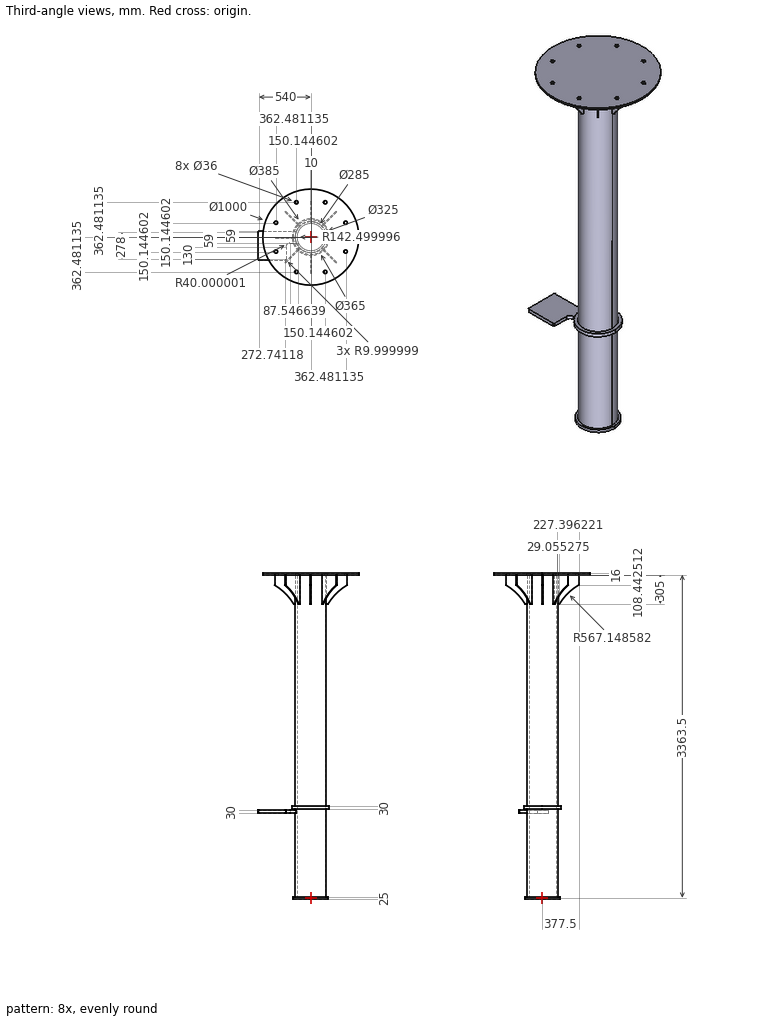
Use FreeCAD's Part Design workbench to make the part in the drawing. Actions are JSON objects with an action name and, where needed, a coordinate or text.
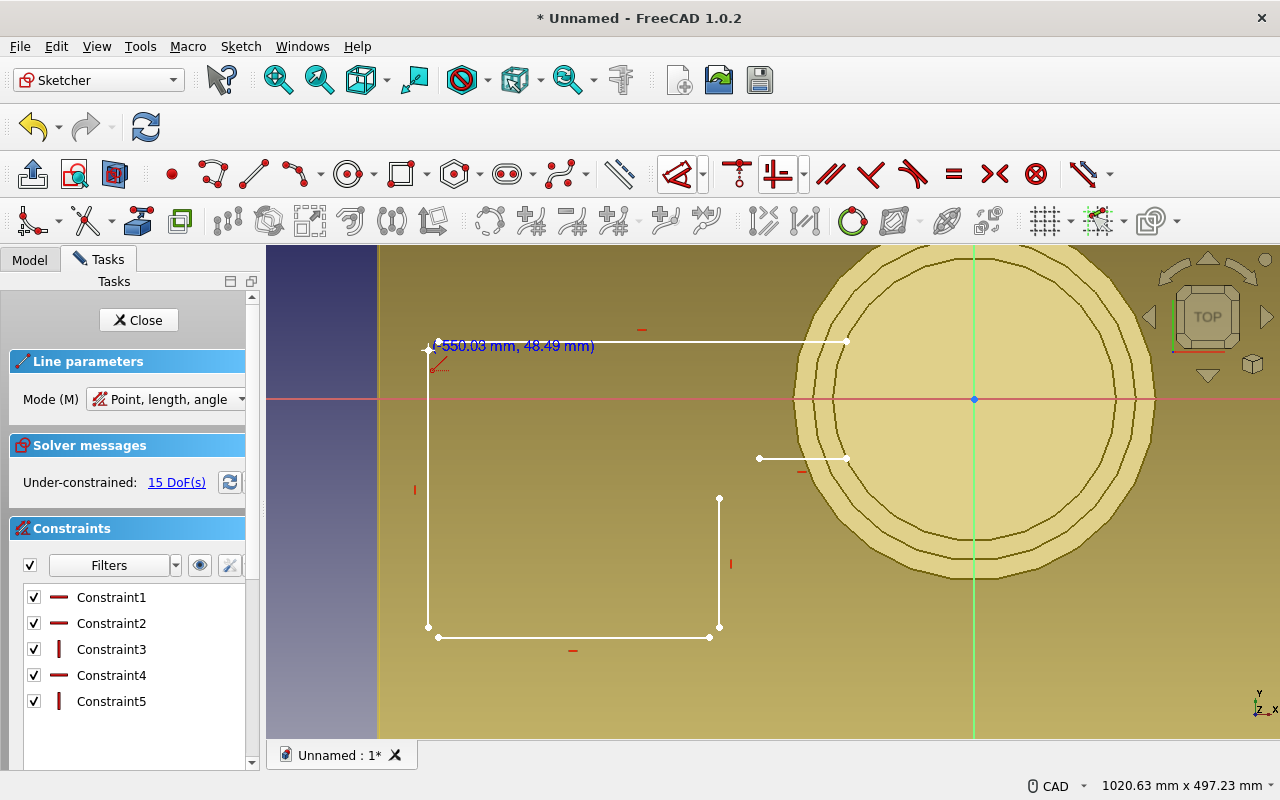
{"action": "key", "text": "g 3 a"}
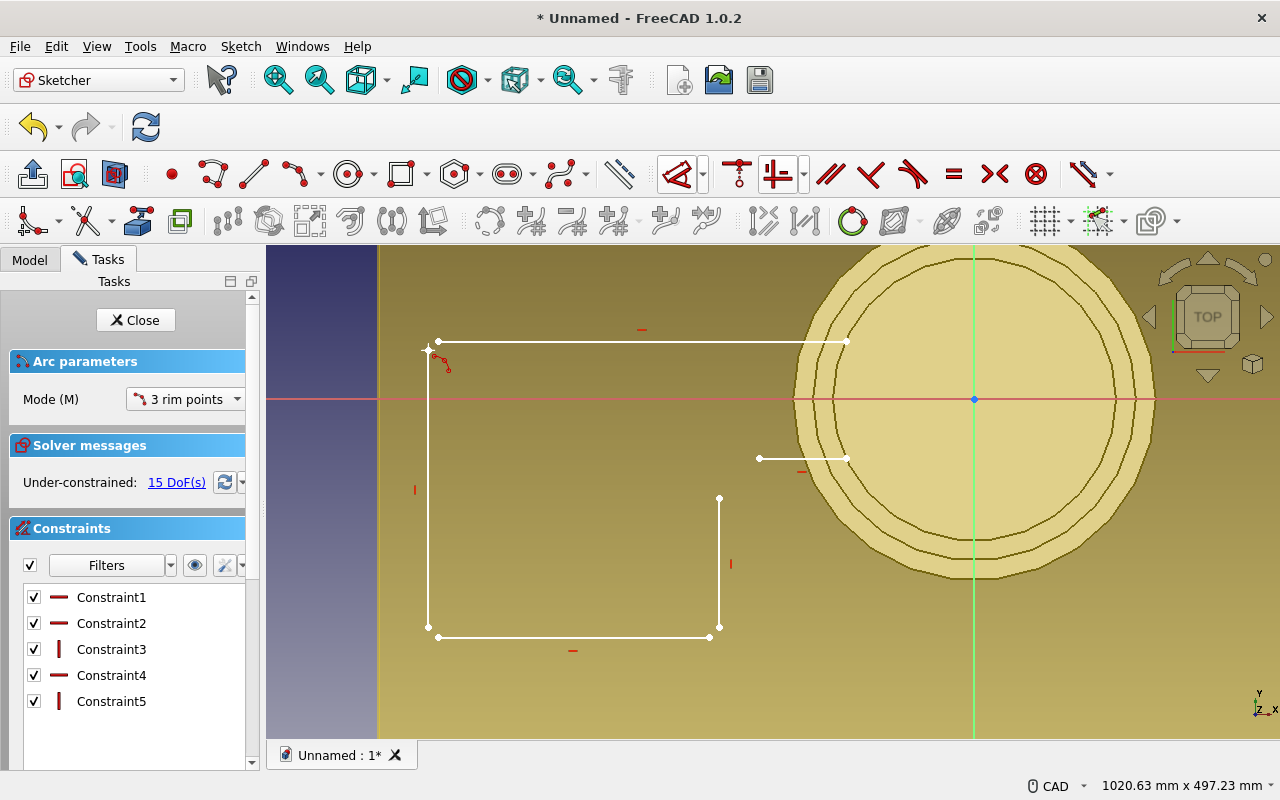
{"action": "left_click", "coordinate": [846, 342]}
{"action": "left_click", "coordinate": [846, 459]}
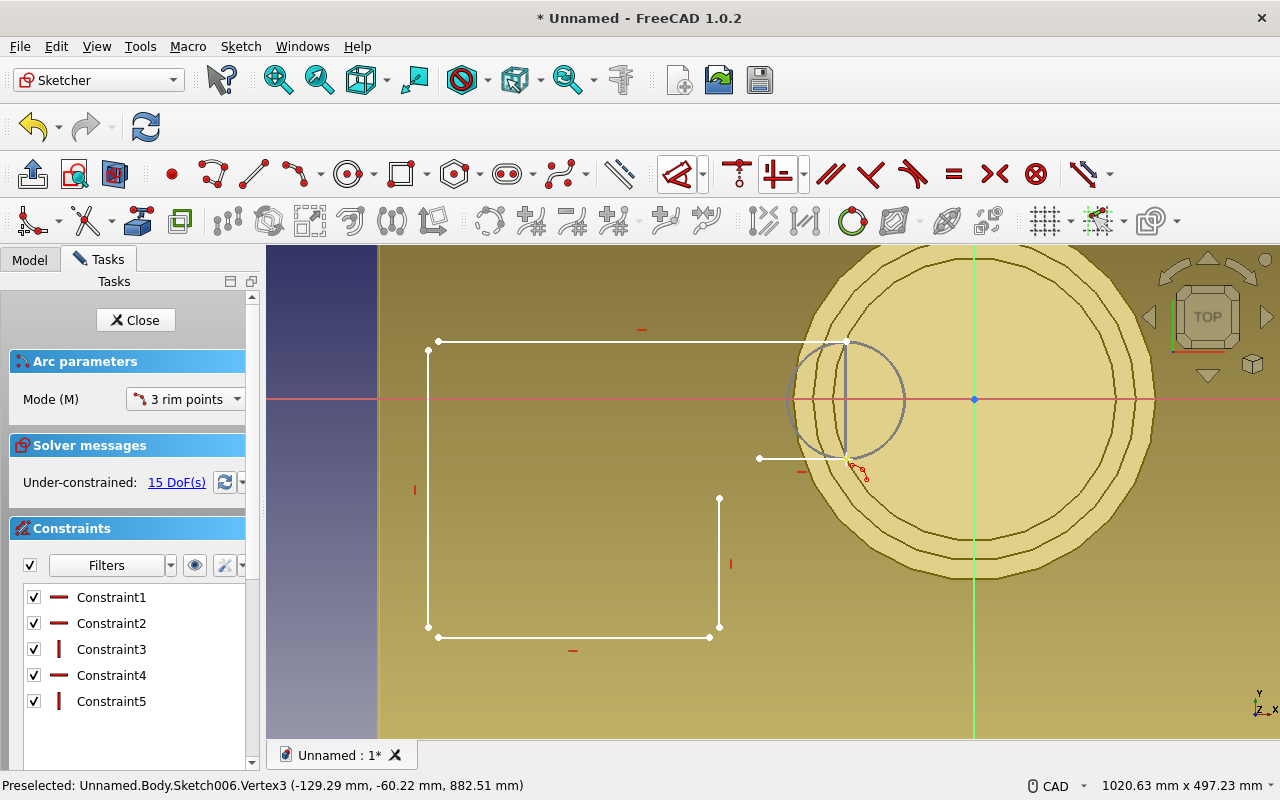
{"action": "scroll", "coordinate": [833, 387], "scroll_direction": "up", "scroll_amount": 2}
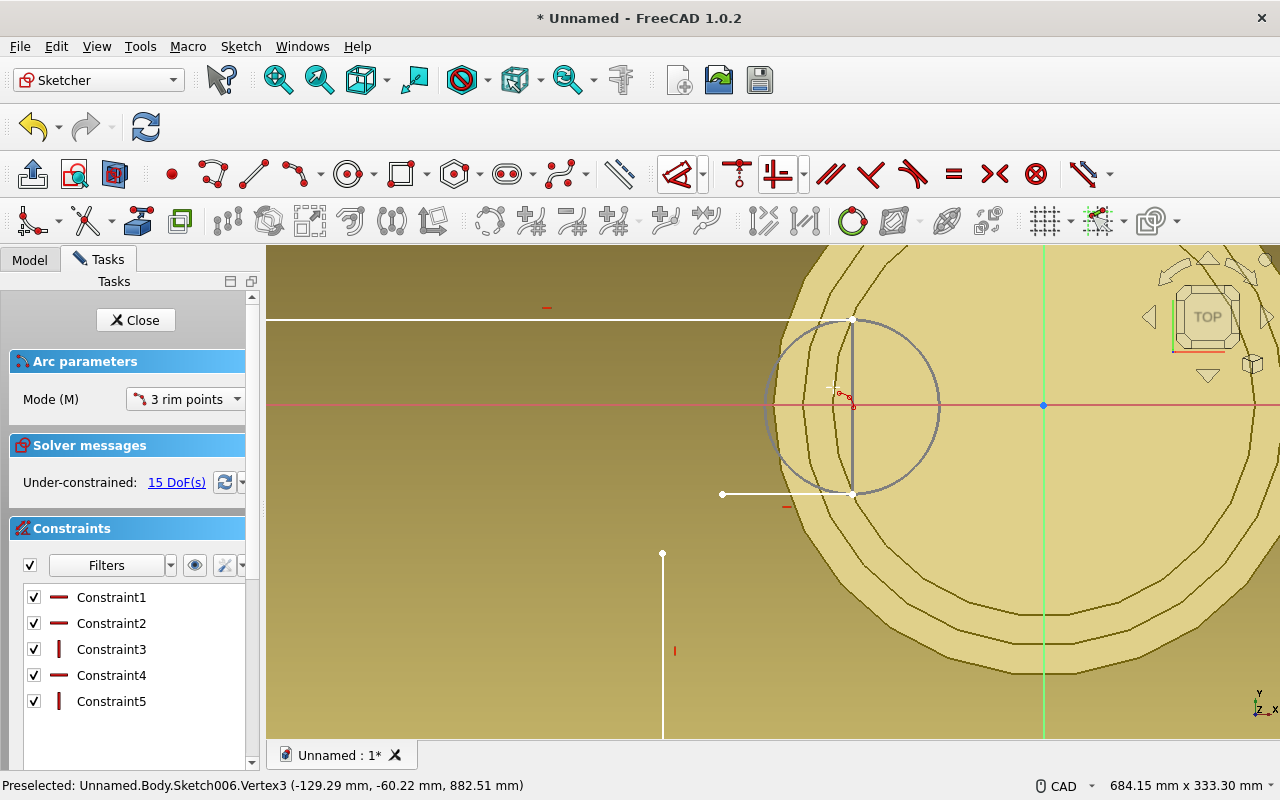
{"action": "left_click", "coordinate": [833, 387]}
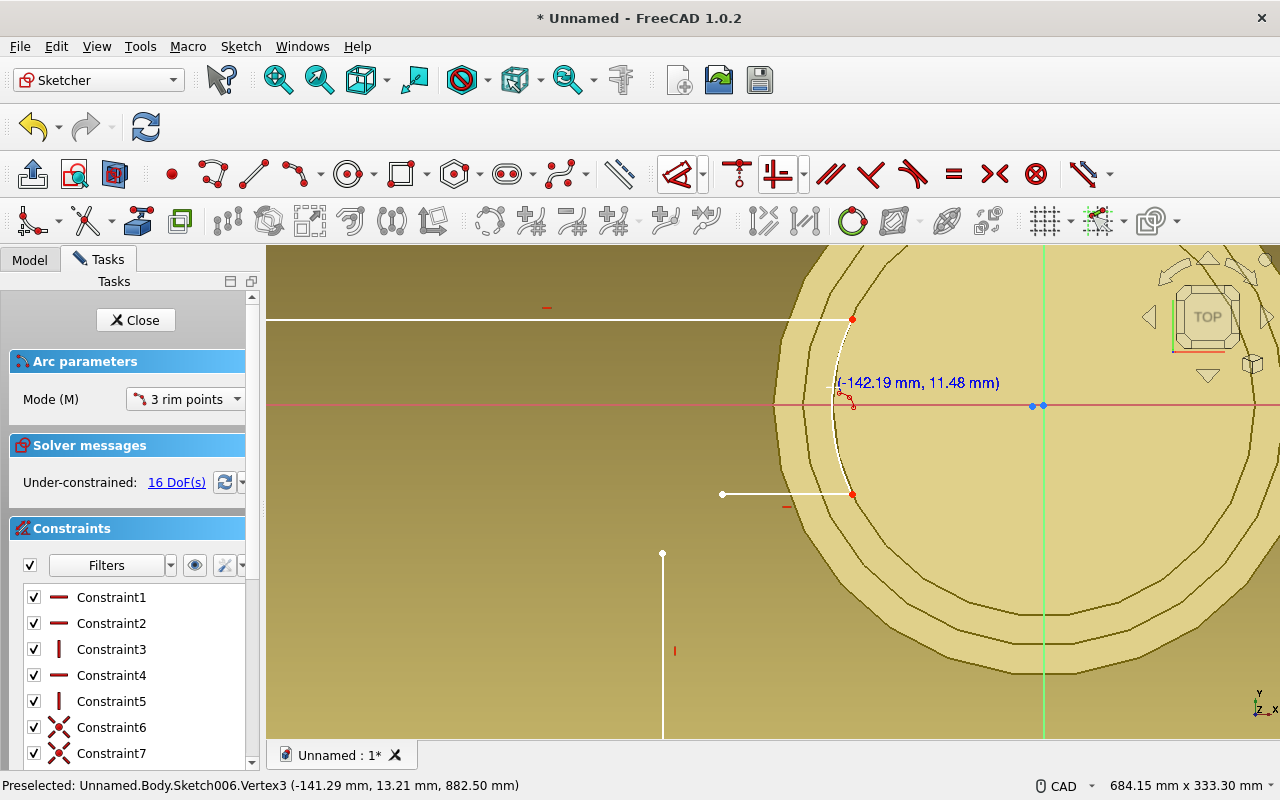
{"action": "left_click", "coordinate": [722, 494]}
{"action": "left_click", "coordinate": [663, 554]}
{"action": "left_click", "coordinate": [680, 510]}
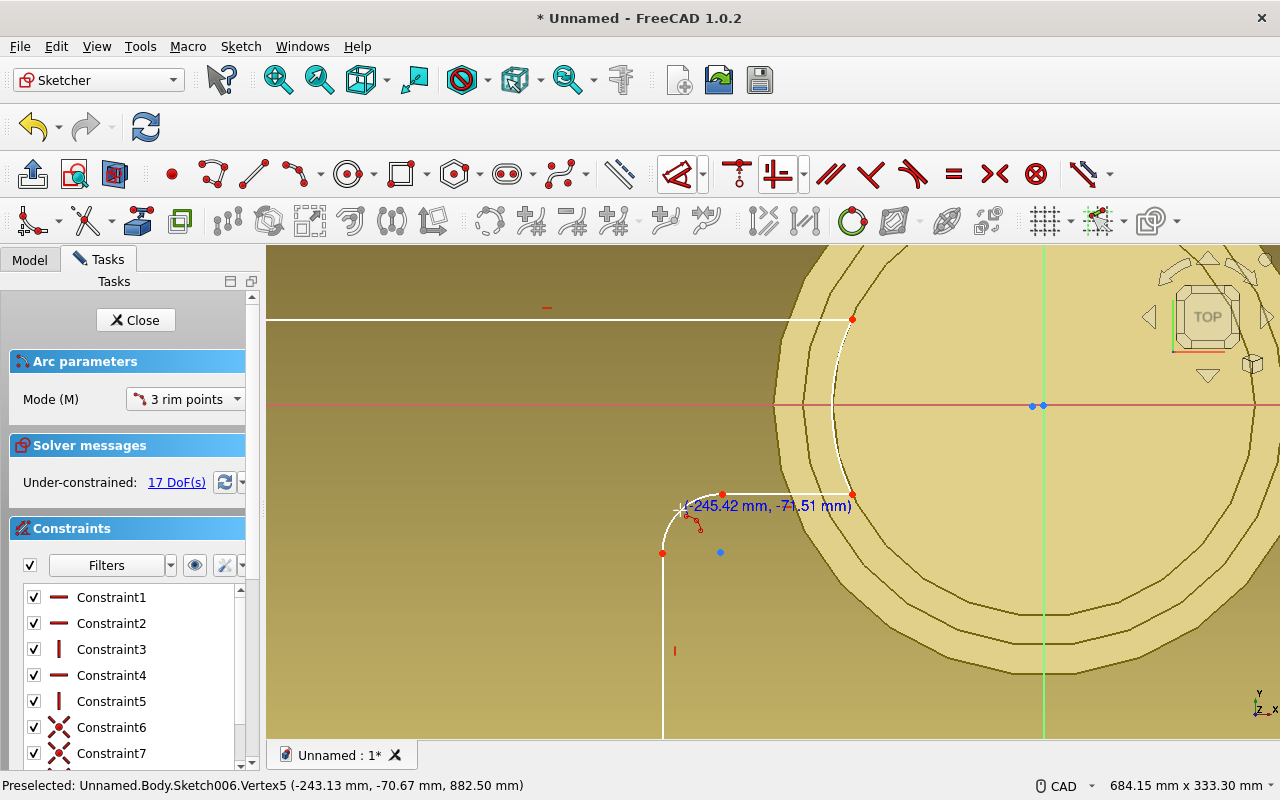
{"action": "scroll", "coordinate": [843, 398], "scroll_direction": "down", "scroll_amount": 2}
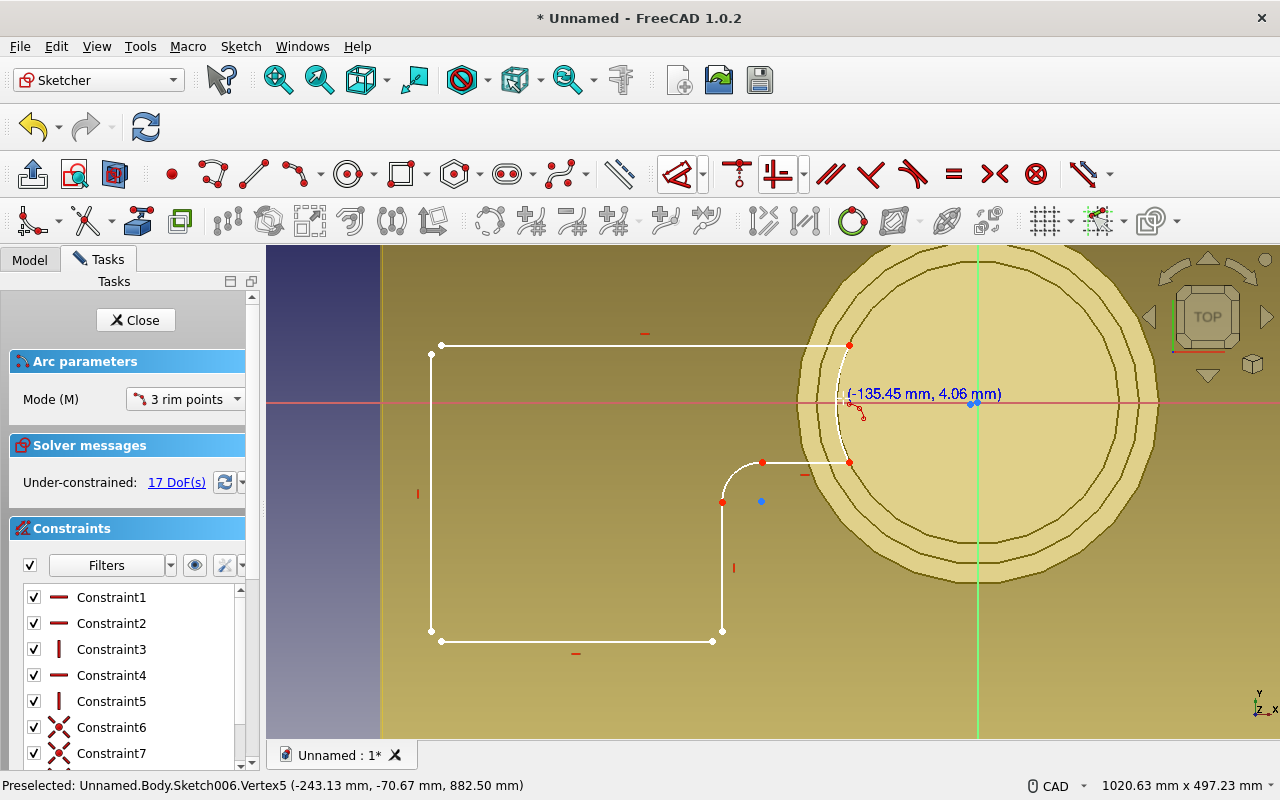
{"action": "left_click", "coordinate": [722, 632]}
{"action": "left_click", "coordinate": [712, 642]}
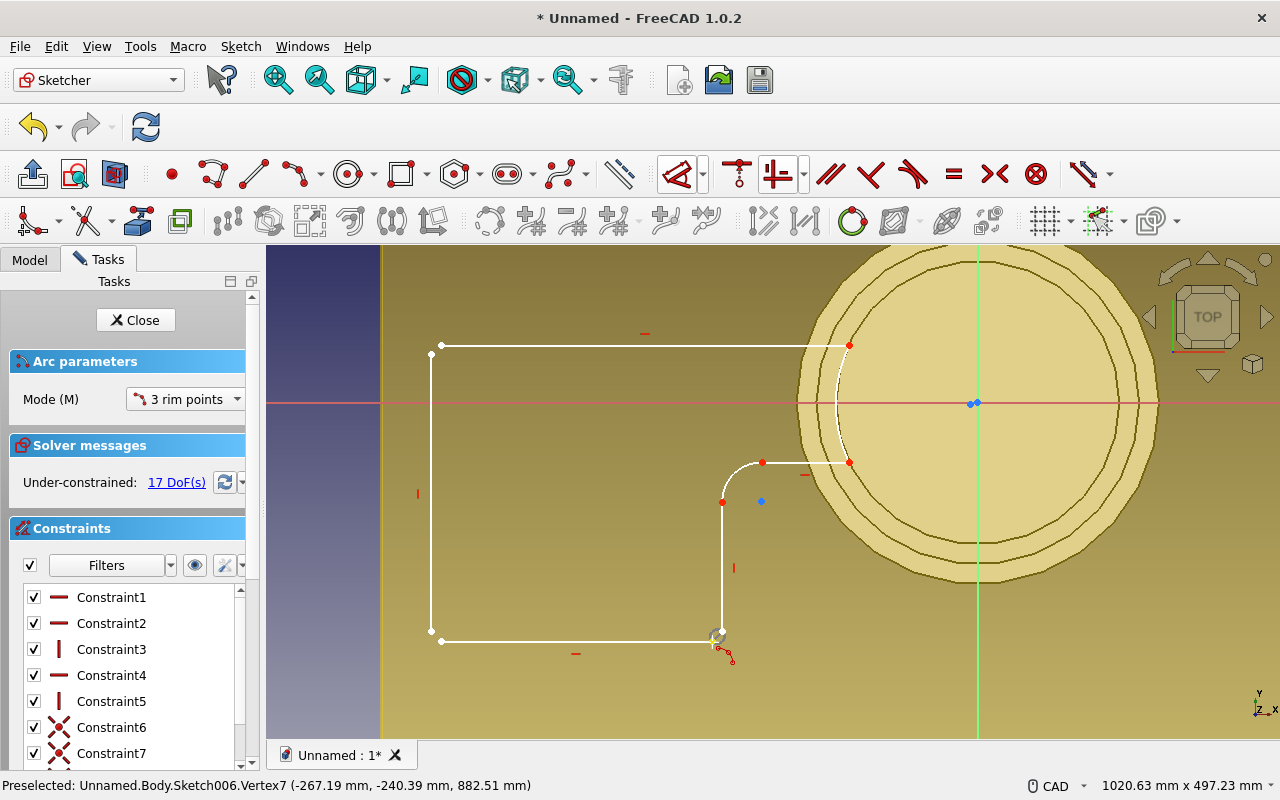
{"action": "scroll", "coordinate": [719, 637], "scroll_direction": "up", "scroll_amount": 9}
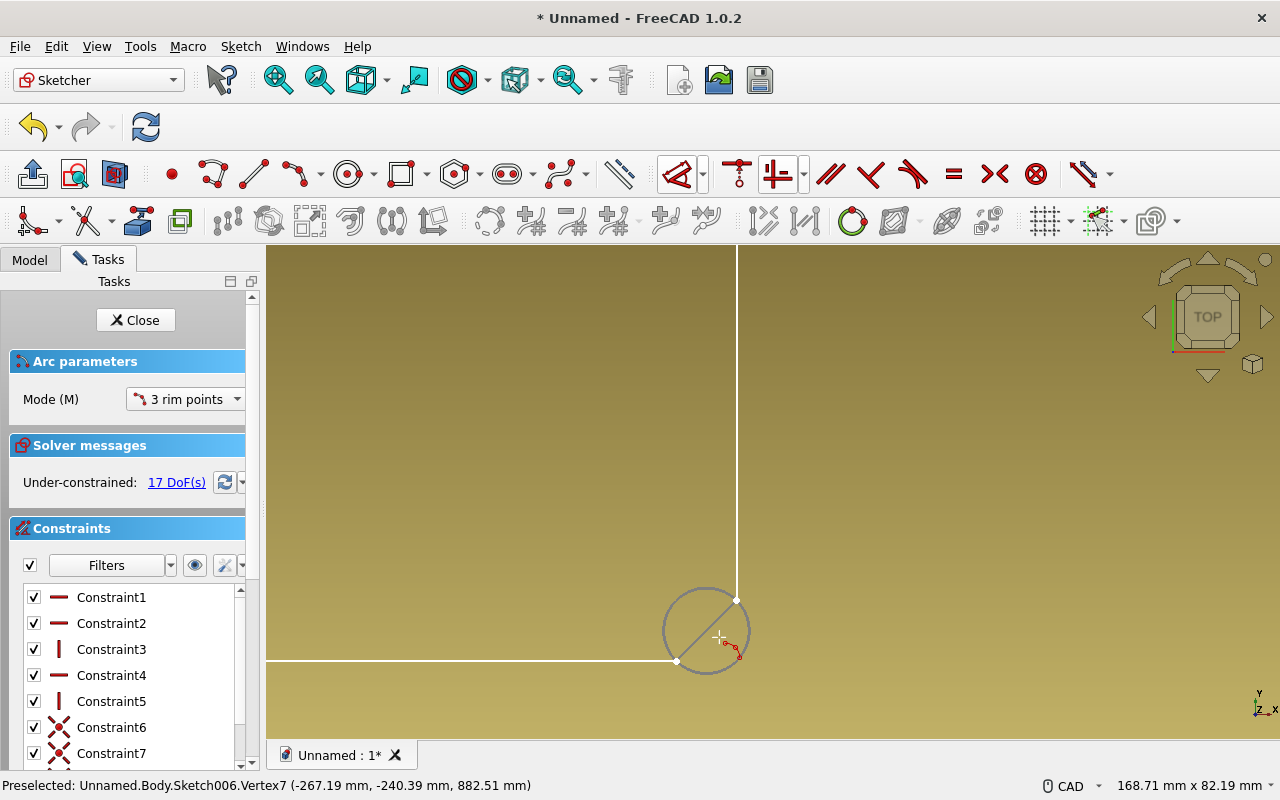
{"action": "left_click", "coordinate": [718, 635]}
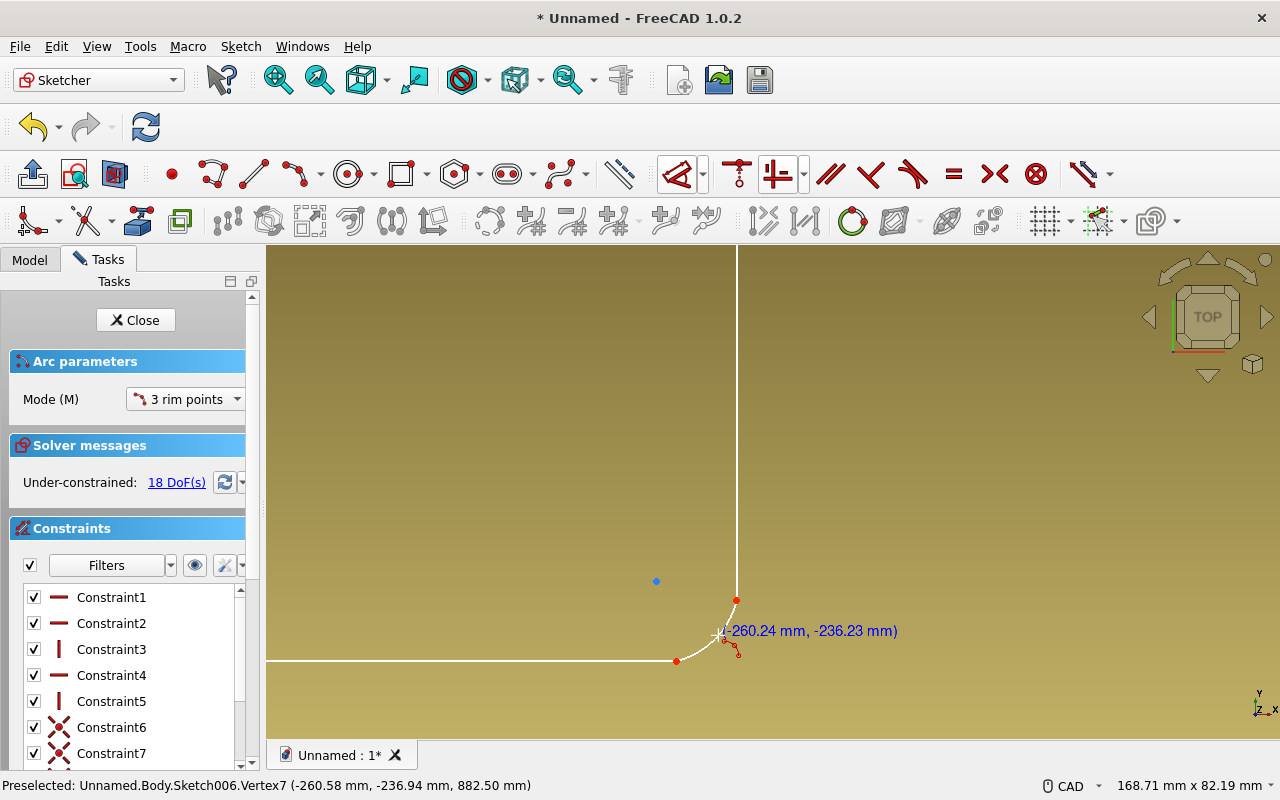
{"action": "scroll", "coordinate": [719, 638], "scroll_direction": "down", "scroll_amount": 9}